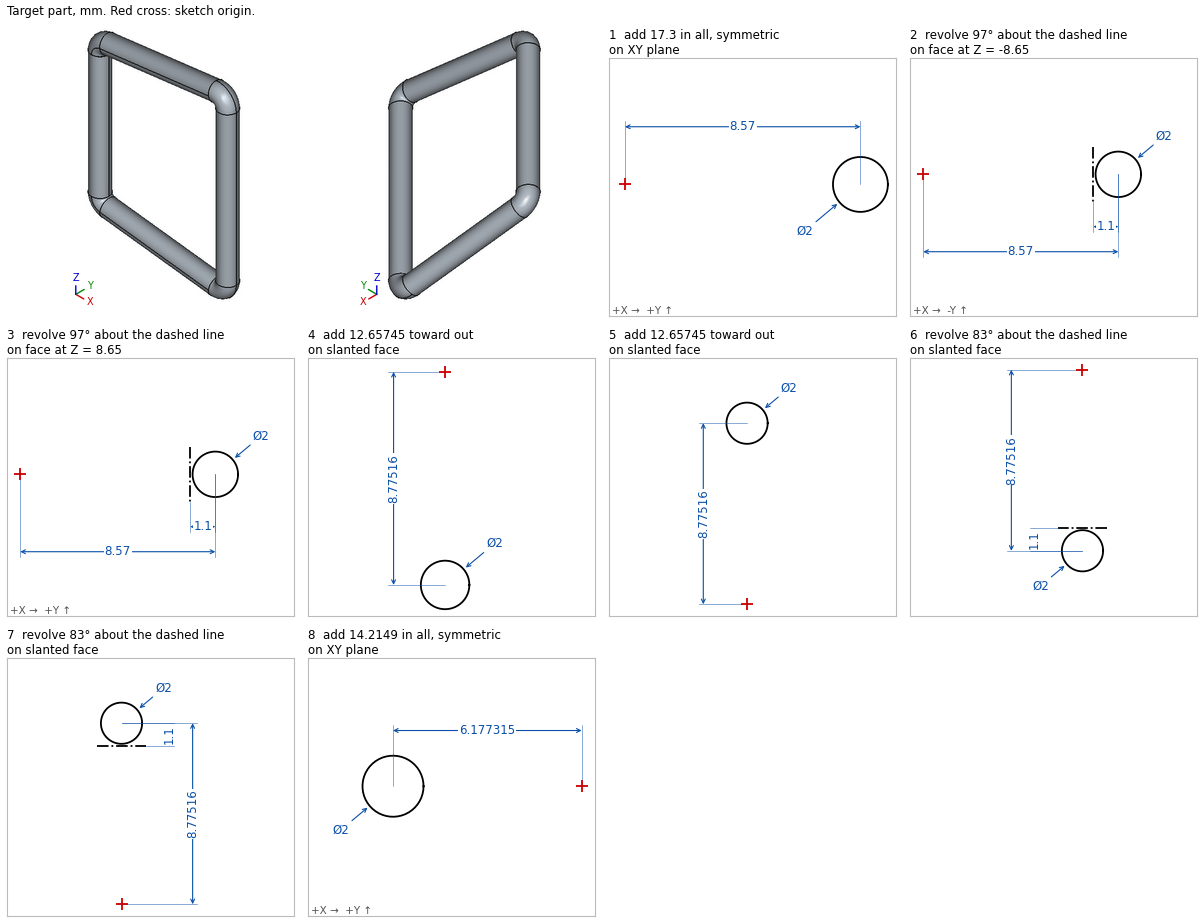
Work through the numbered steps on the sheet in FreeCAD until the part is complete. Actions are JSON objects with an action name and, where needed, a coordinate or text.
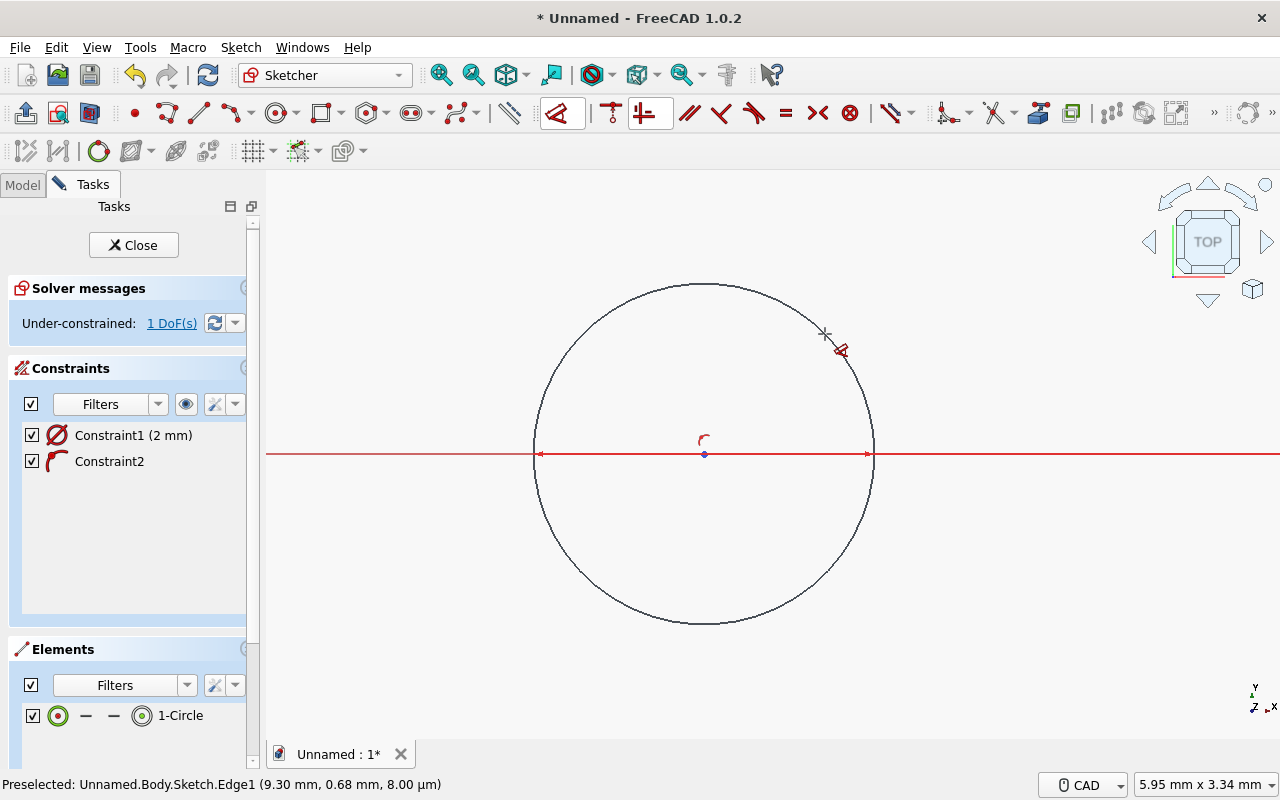
{"action": "left_click", "coordinate": [704, 454]}
{"action": "left_click", "coordinate": [499, 488]}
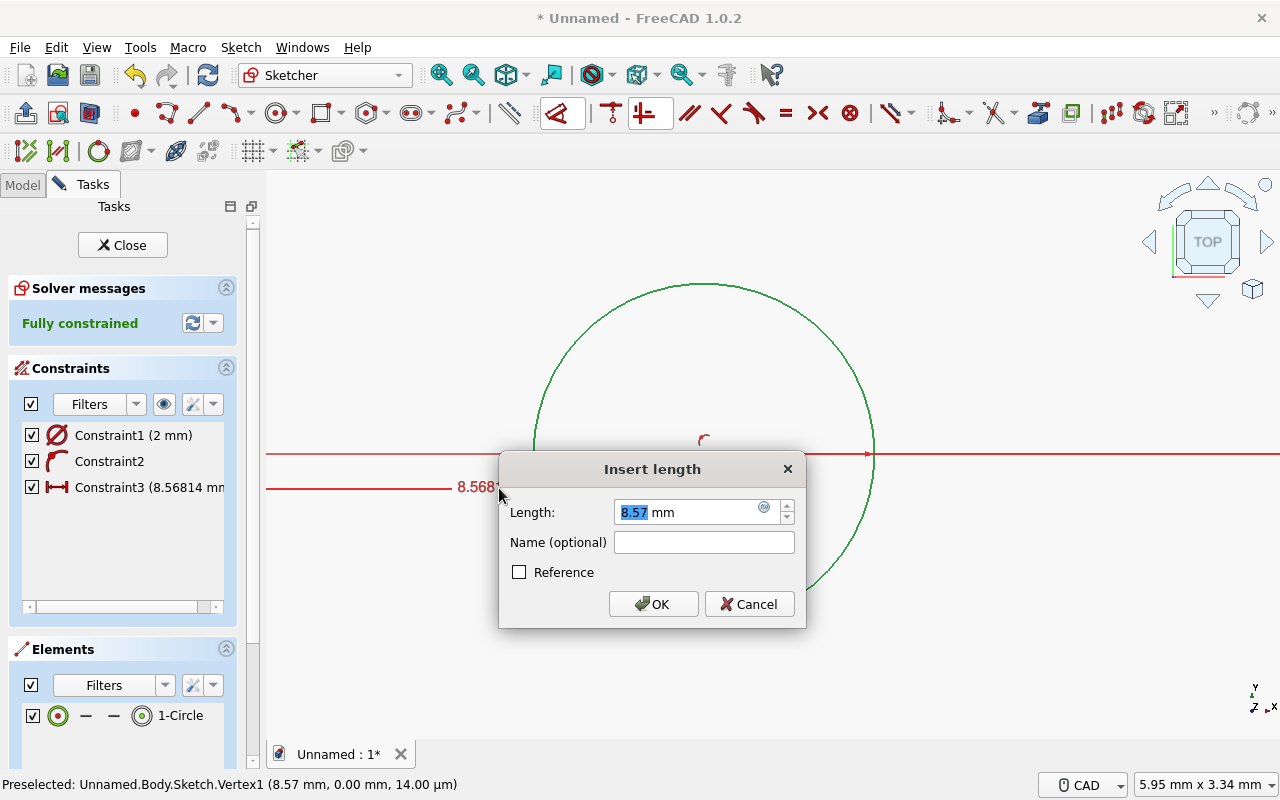
{"action": "type", "text": "8.57"}
{"action": "key", "text": "Return"}
{"action": "key", "text": "Escape"}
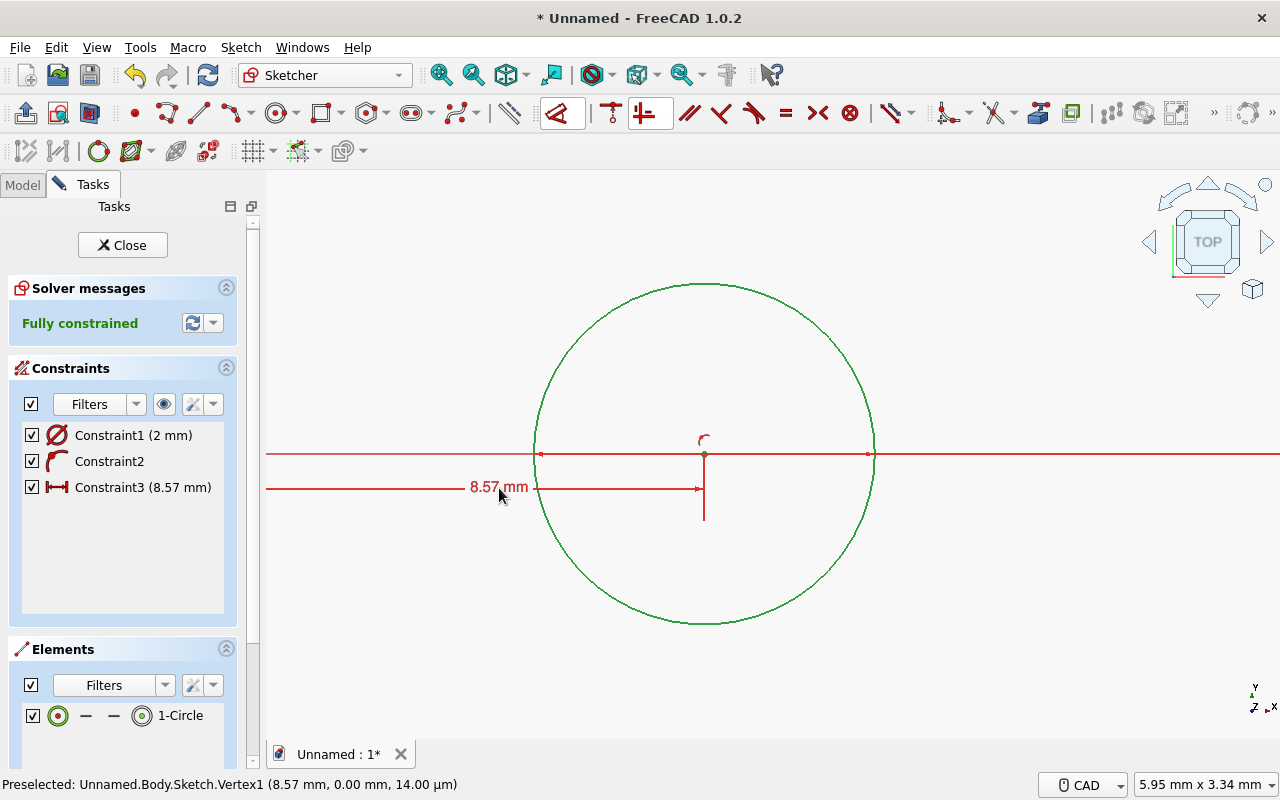
{"action": "left_click", "coordinate": [123, 245]}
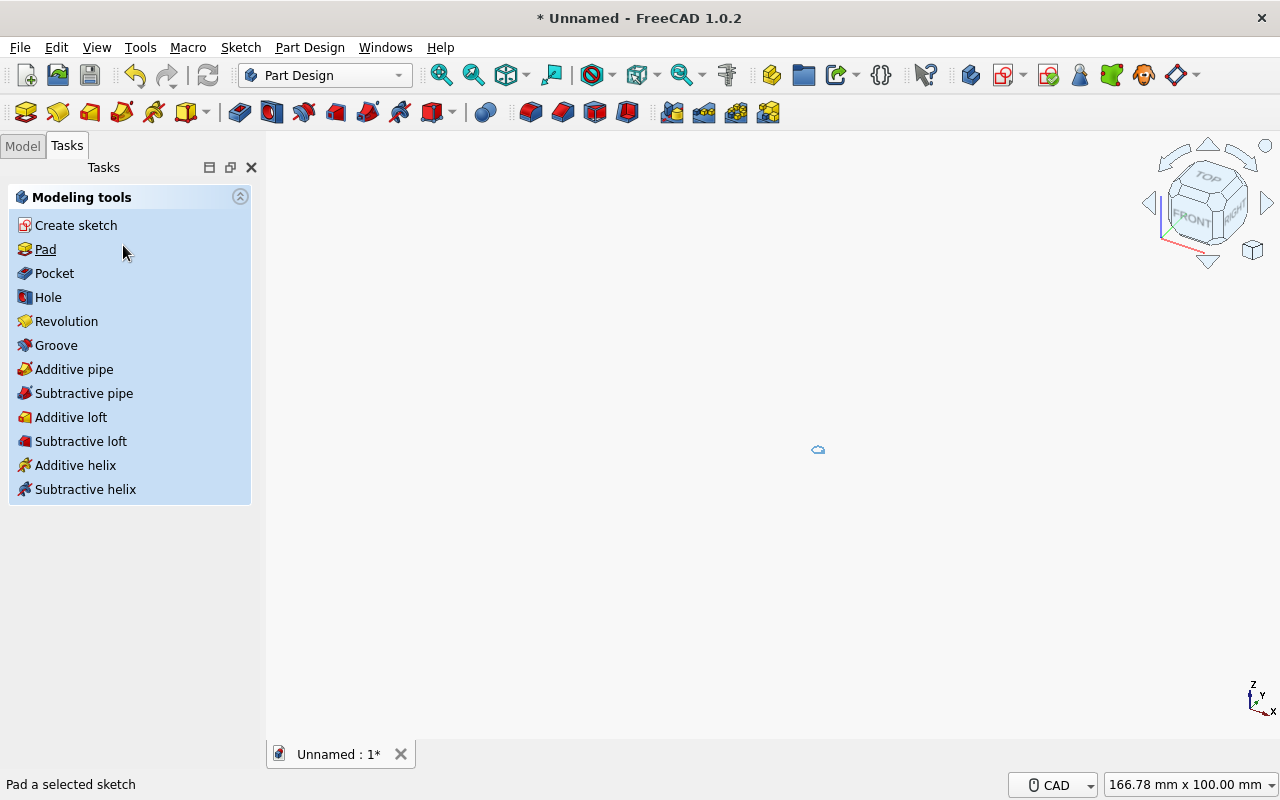
{"action": "left_click", "coordinate": [26, 112]}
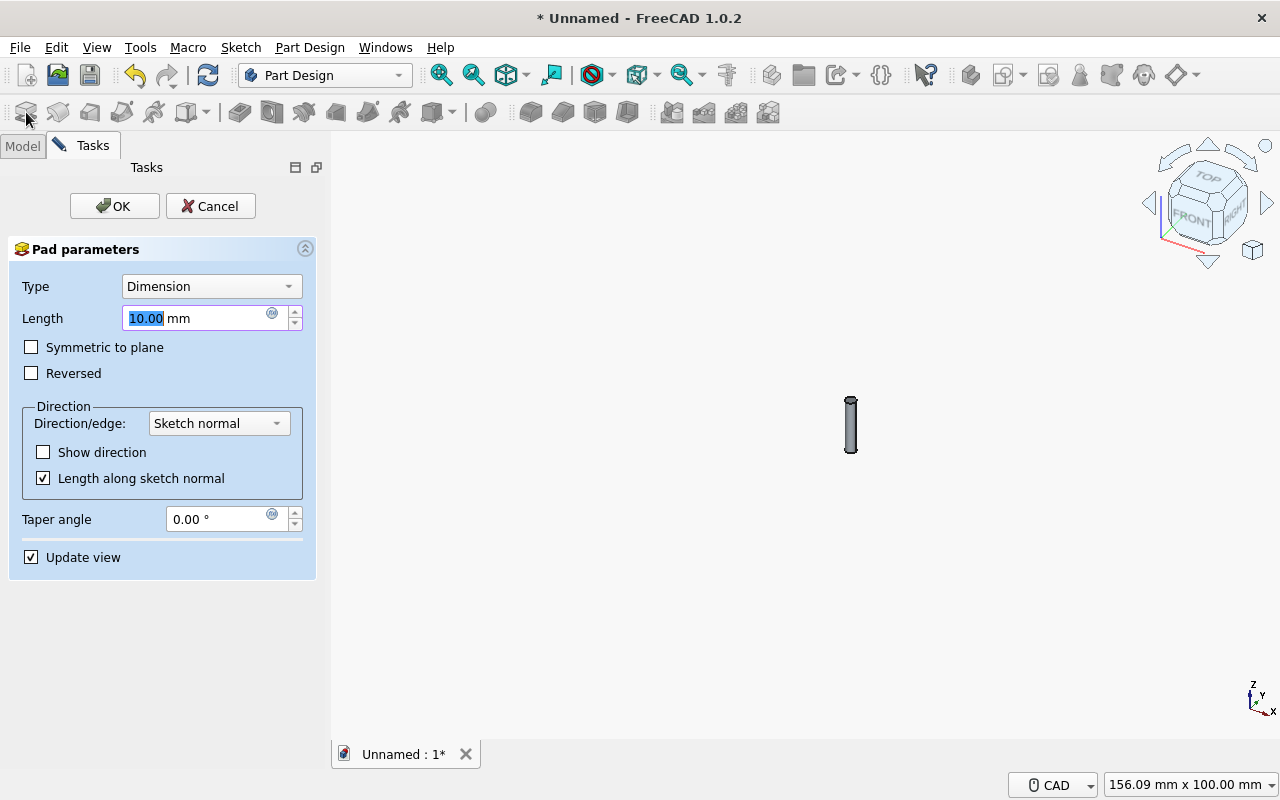
{"action": "type", "text": "17.3"}
{"action": "key", "text": "Tab"}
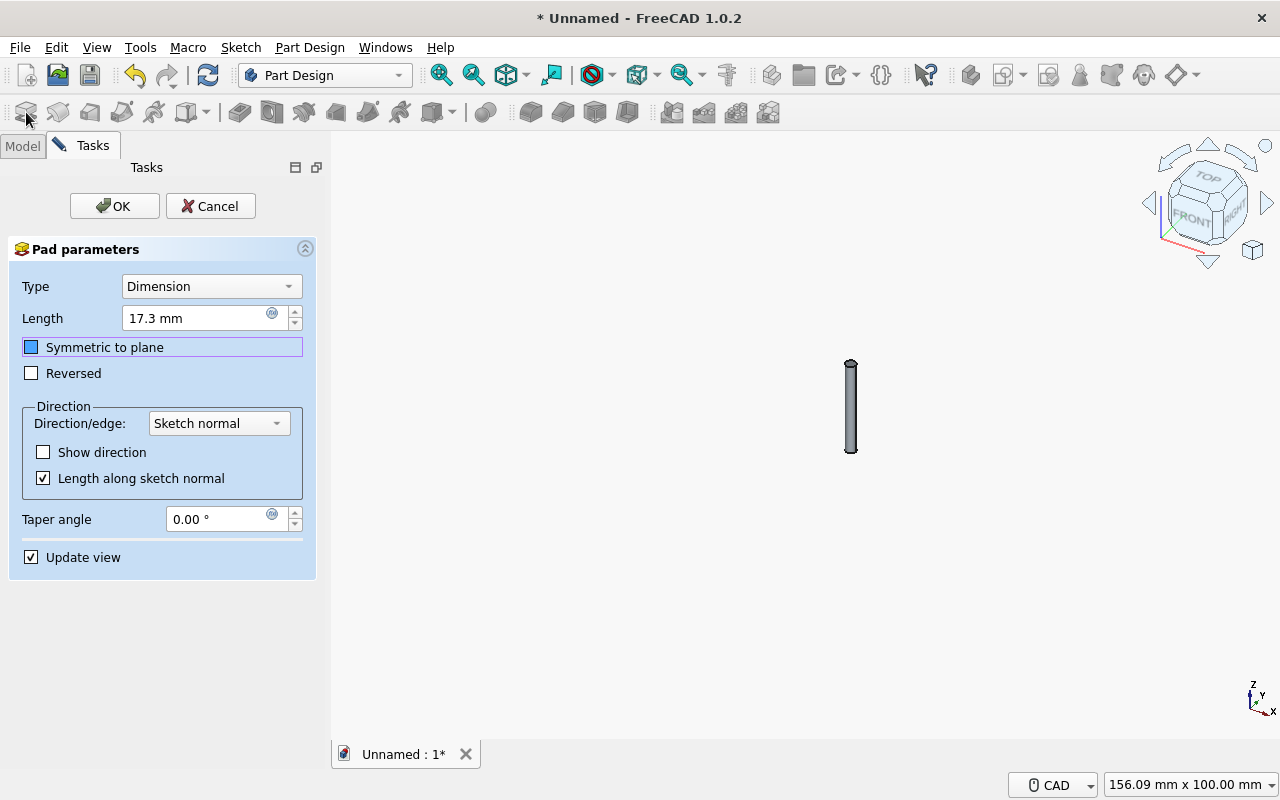
{"action": "left_click", "coordinate": [30, 347]}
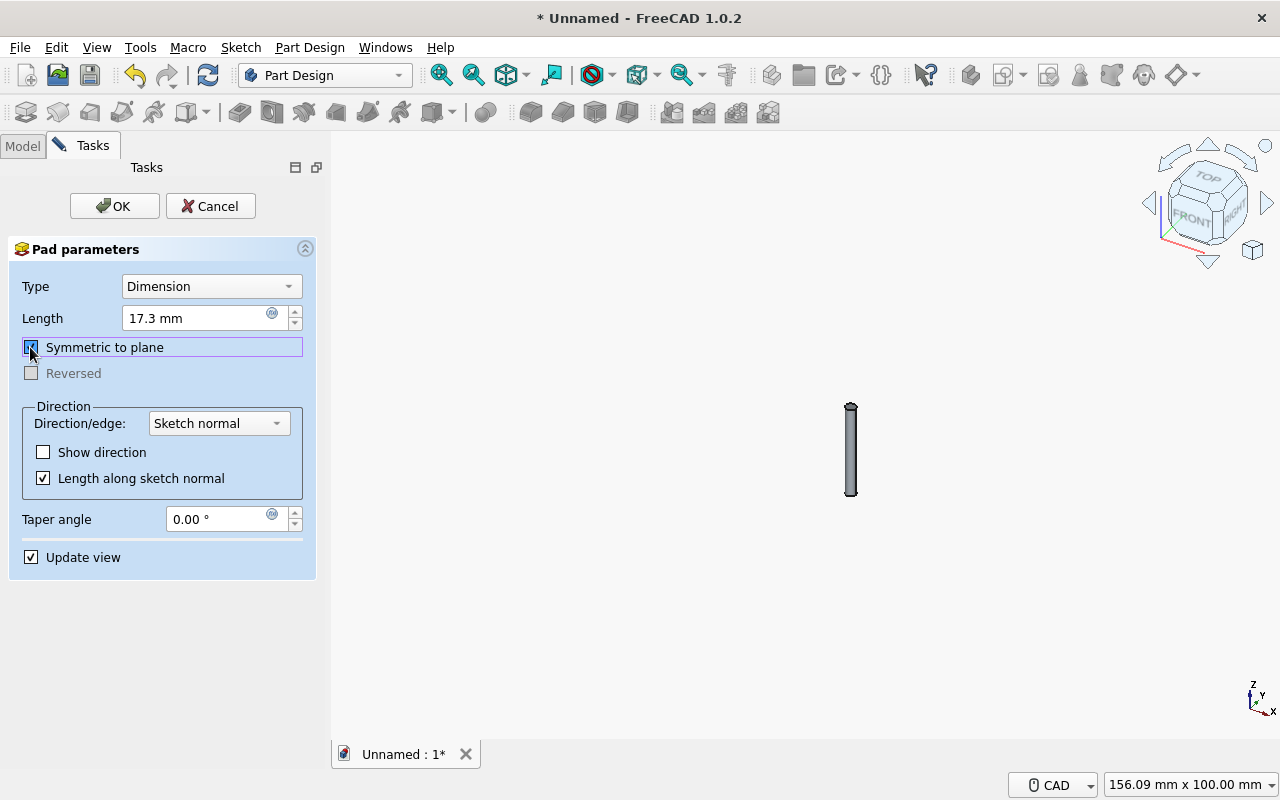
{"action": "left_click", "coordinate": [115, 206]}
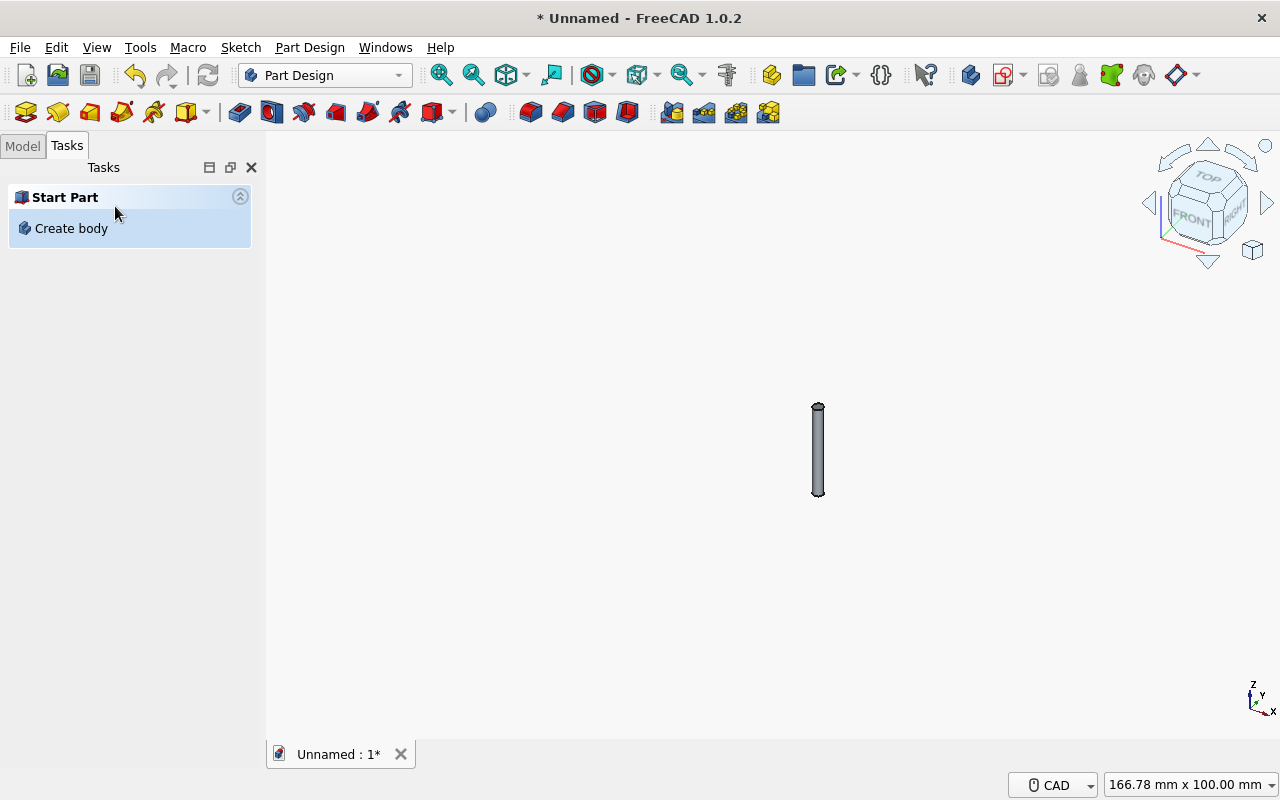
{"action": "left_click", "coordinate": [442, 76]}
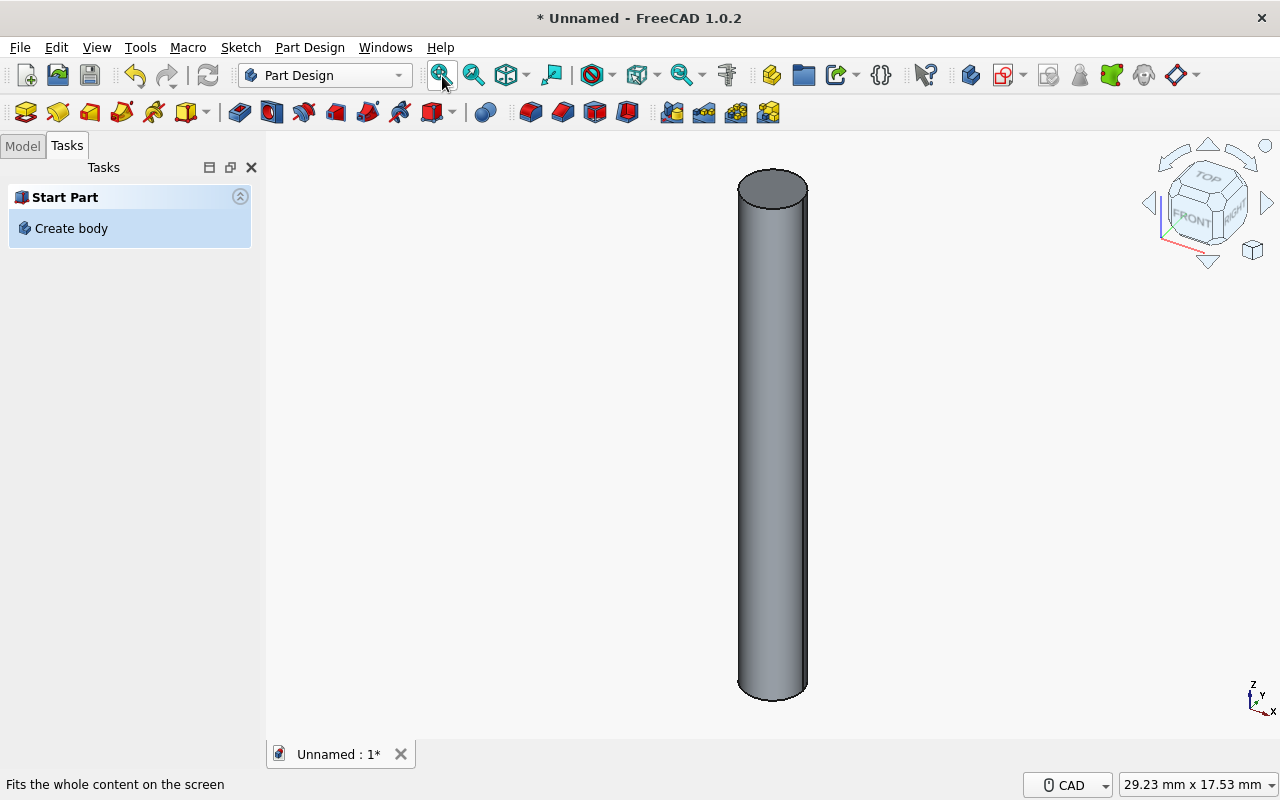
{"action": "key", "text": "5"}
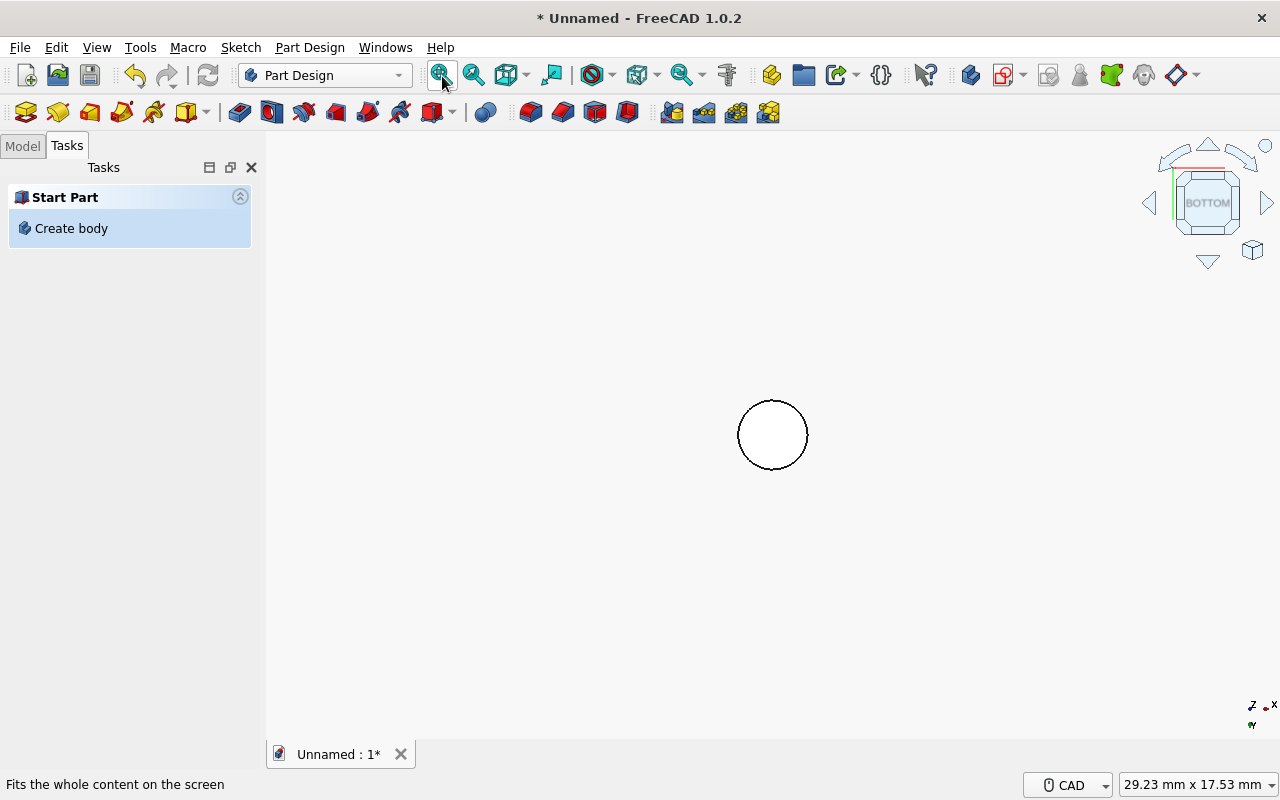
{"action": "left_click", "coordinate": [442, 76]}